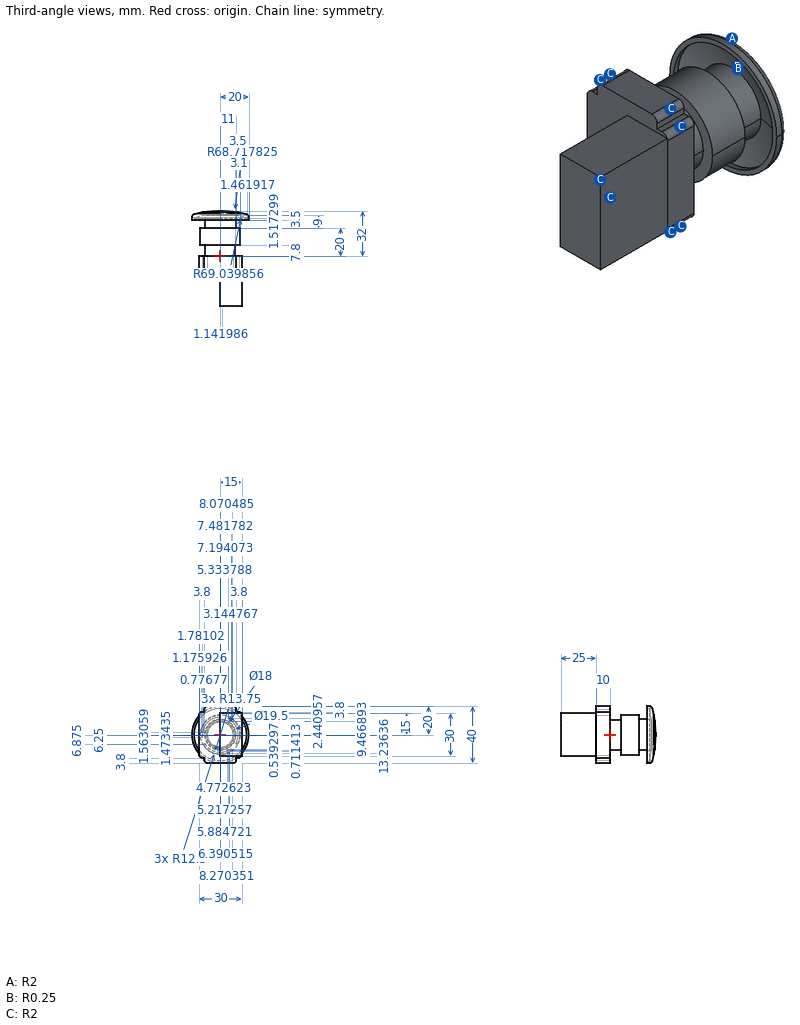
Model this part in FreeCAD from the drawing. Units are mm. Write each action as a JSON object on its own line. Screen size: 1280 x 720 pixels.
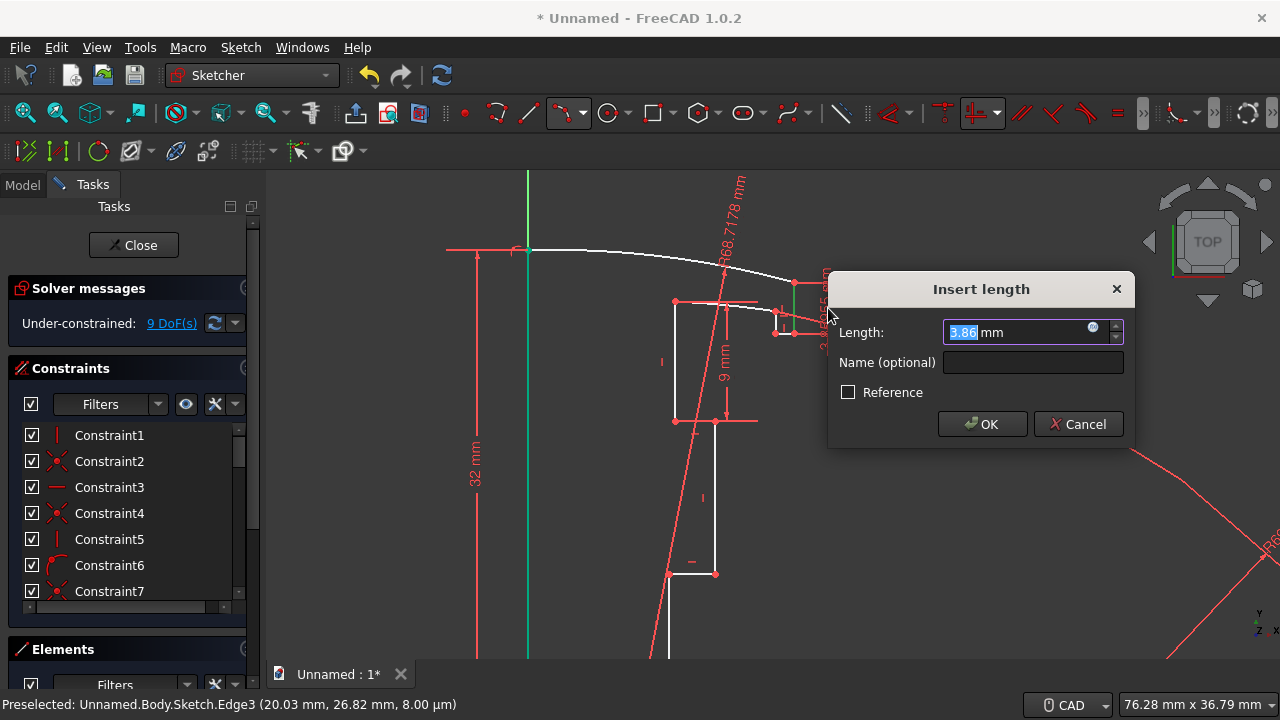
{"action": "type", "text": "3.5"}
{"action": "key", "text": "Return"}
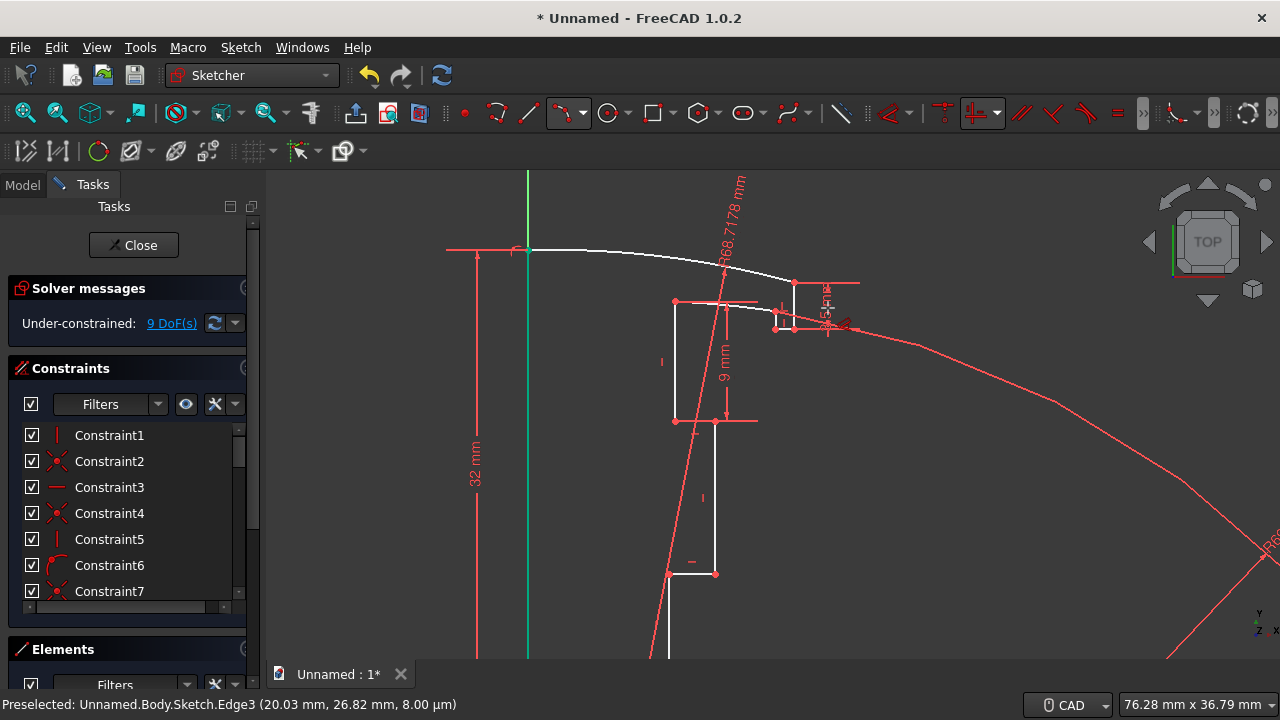
{"action": "left_click", "coordinate": [669, 604]}
{"action": "left_click", "coordinate": [703, 603]}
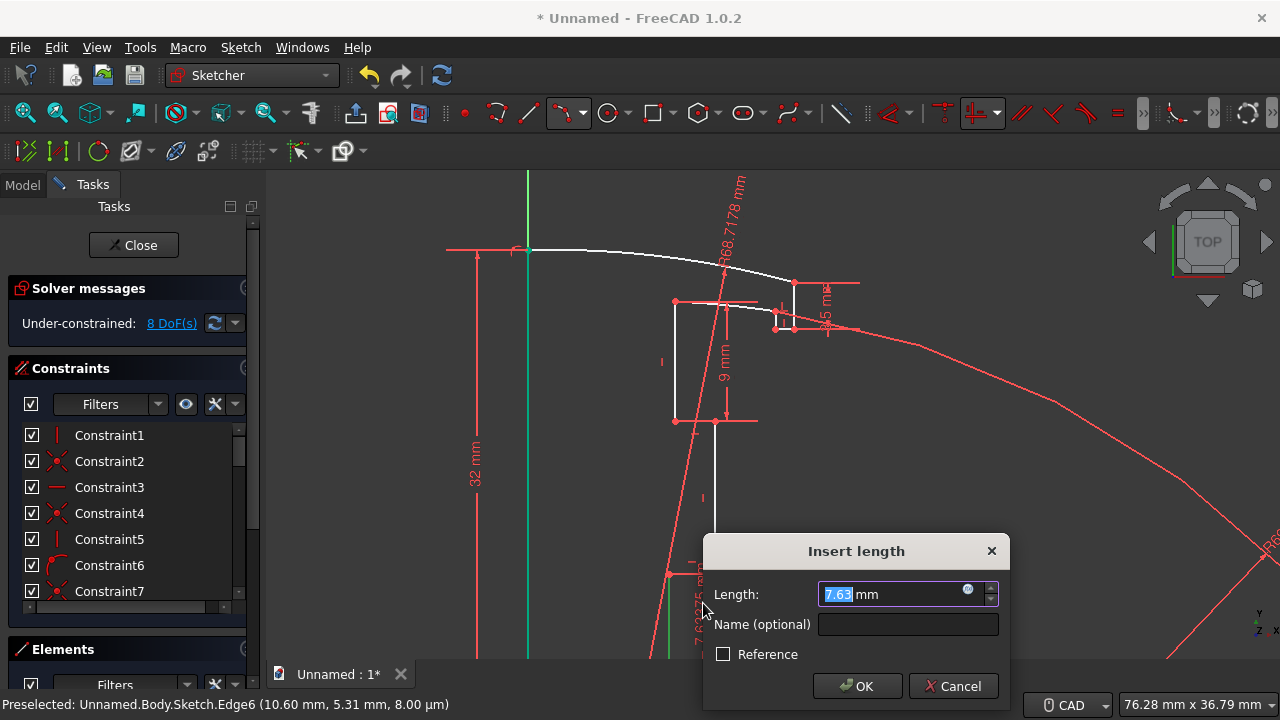
{"action": "type", "text": "7.8"}
{"action": "key", "text": "Return"}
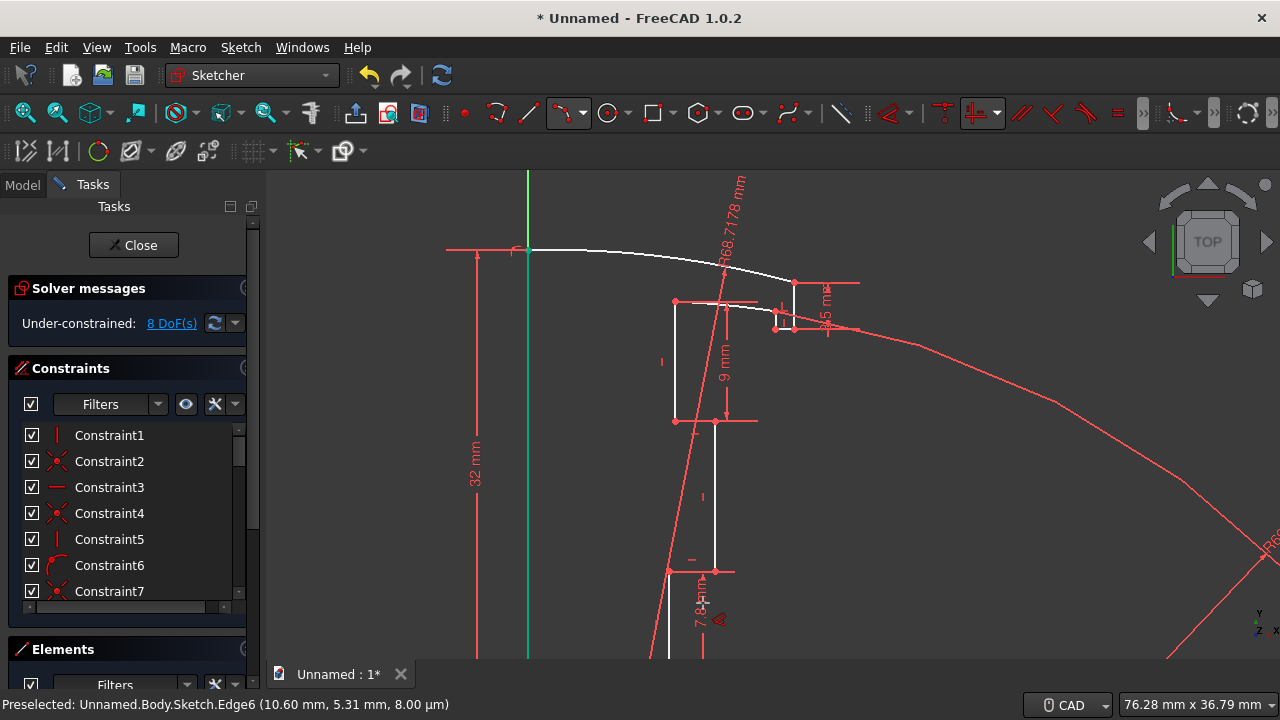
{"action": "left_click", "coordinate": [683, 572]}
{"action": "left_click", "coordinate": [692, 538]}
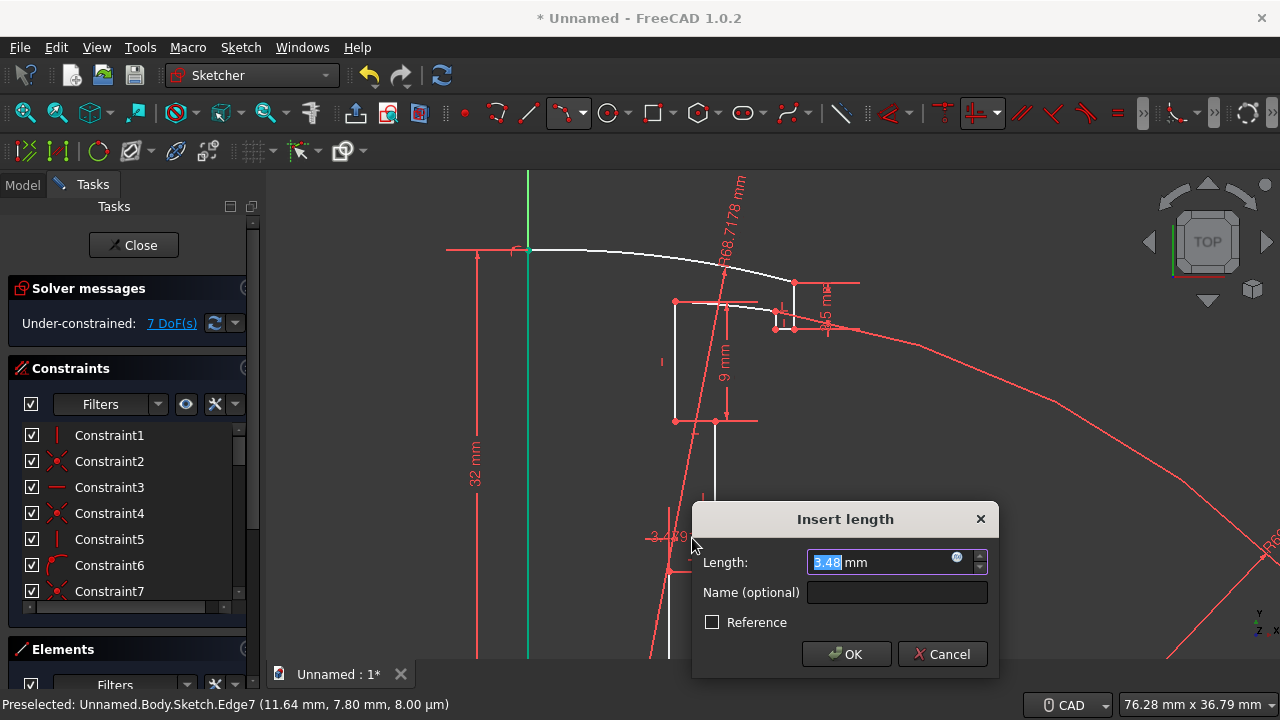
{"action": "type", "text": "3.5"}
{"action": "key", "text": "Return"}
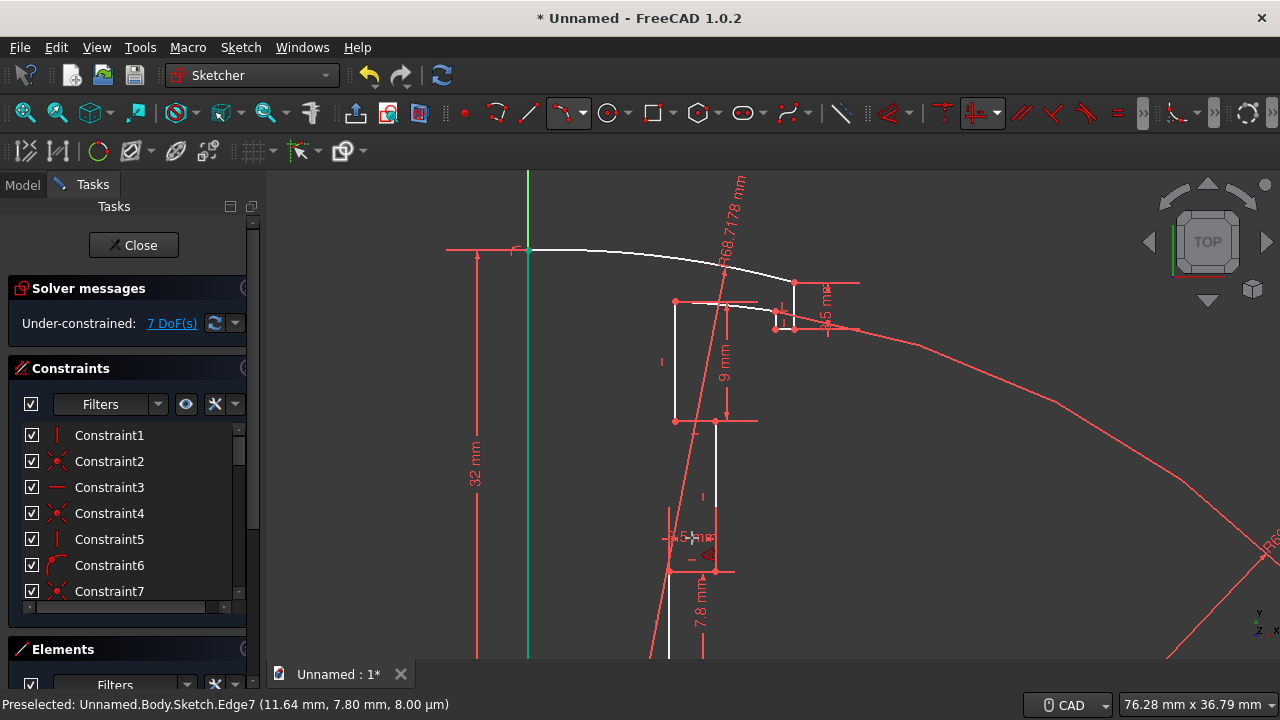
{"action": "left_click", "coordinate": [703, 421]}
{"action": "left_click", "coordinate": [695, 387]}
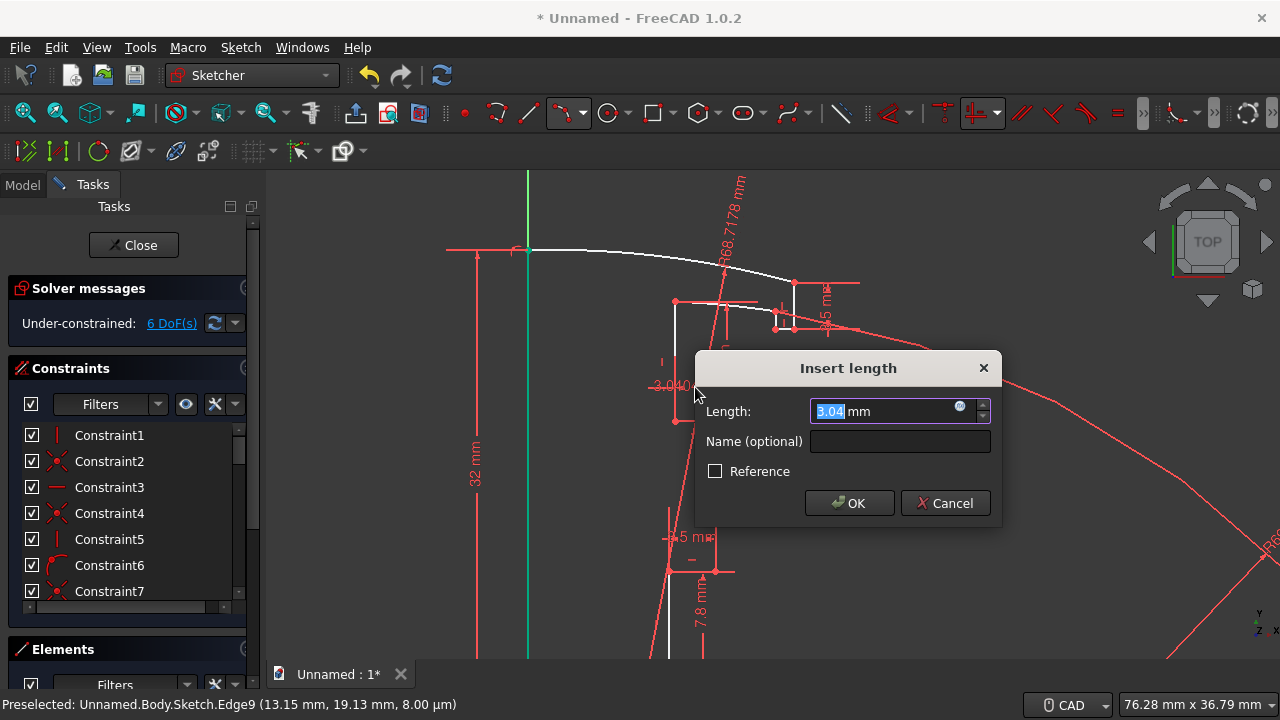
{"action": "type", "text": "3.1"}
{"action": "key", "text": "Return"}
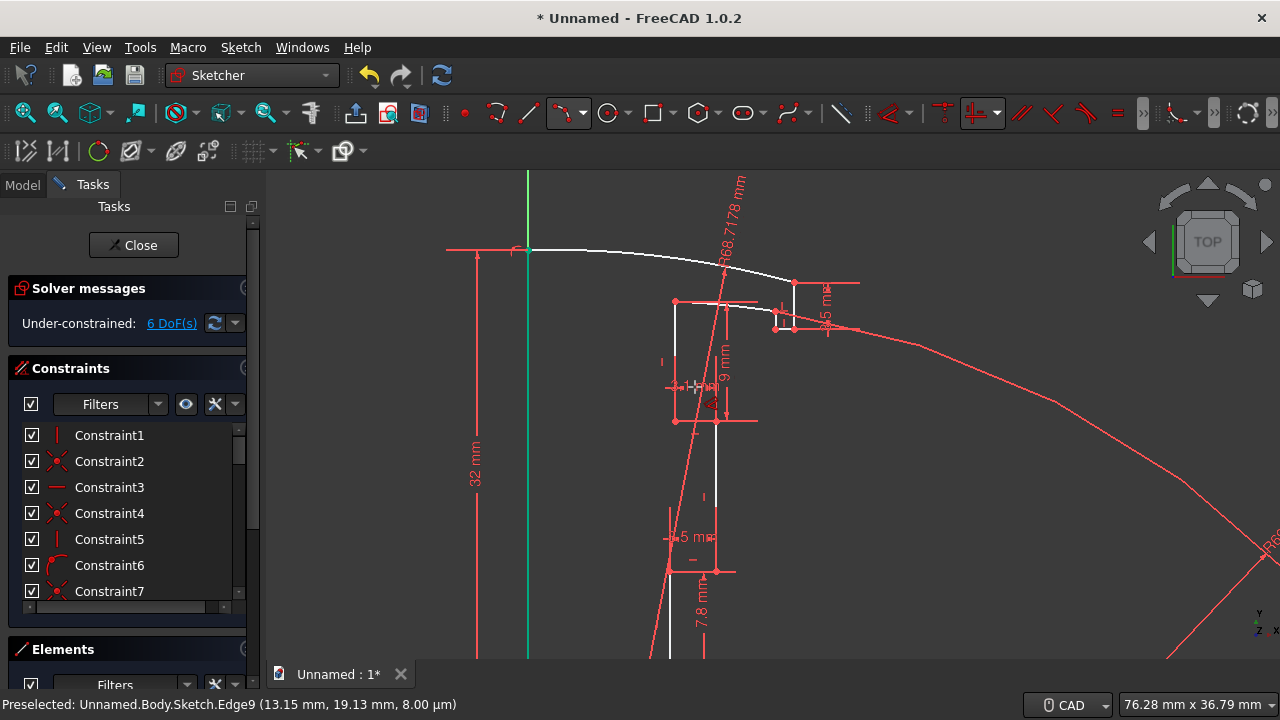
{"action": "left_click", "coordinate": [794, 329]}
{"action": "left_click", "coordinate": [661, 295]}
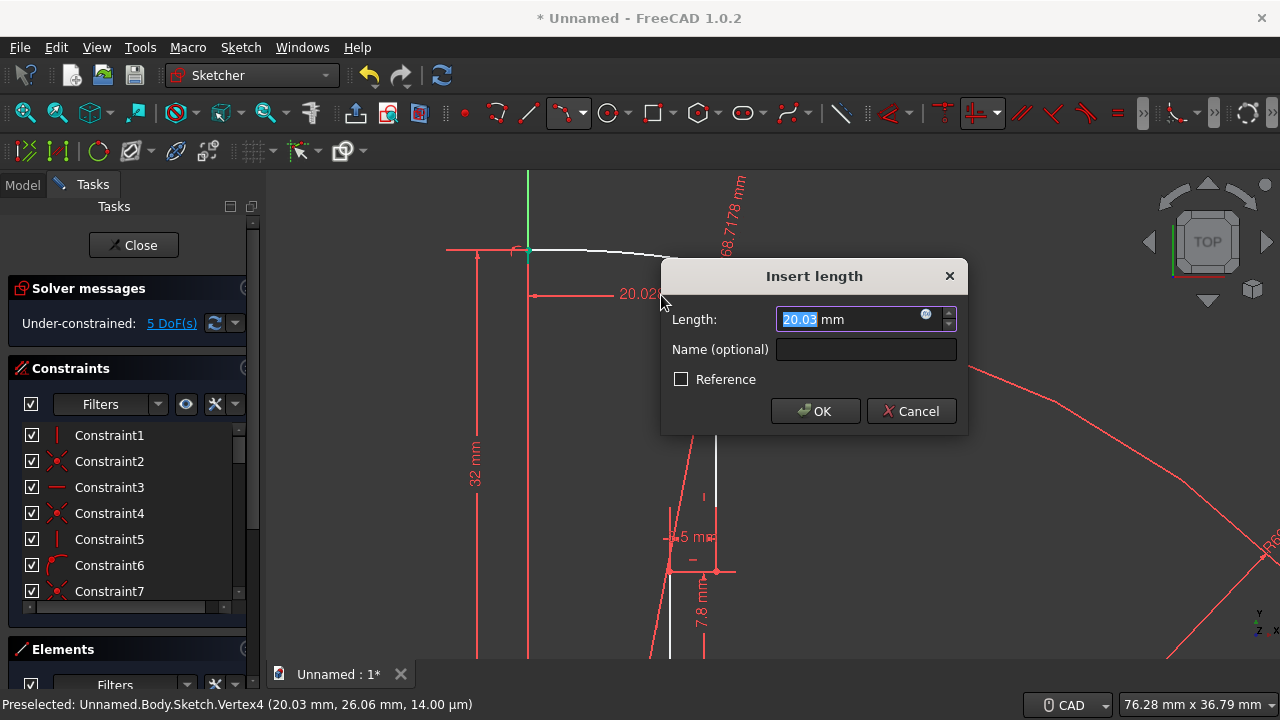
{"action": "type", "text": "20"}
{"action": "key", "text": "Return"}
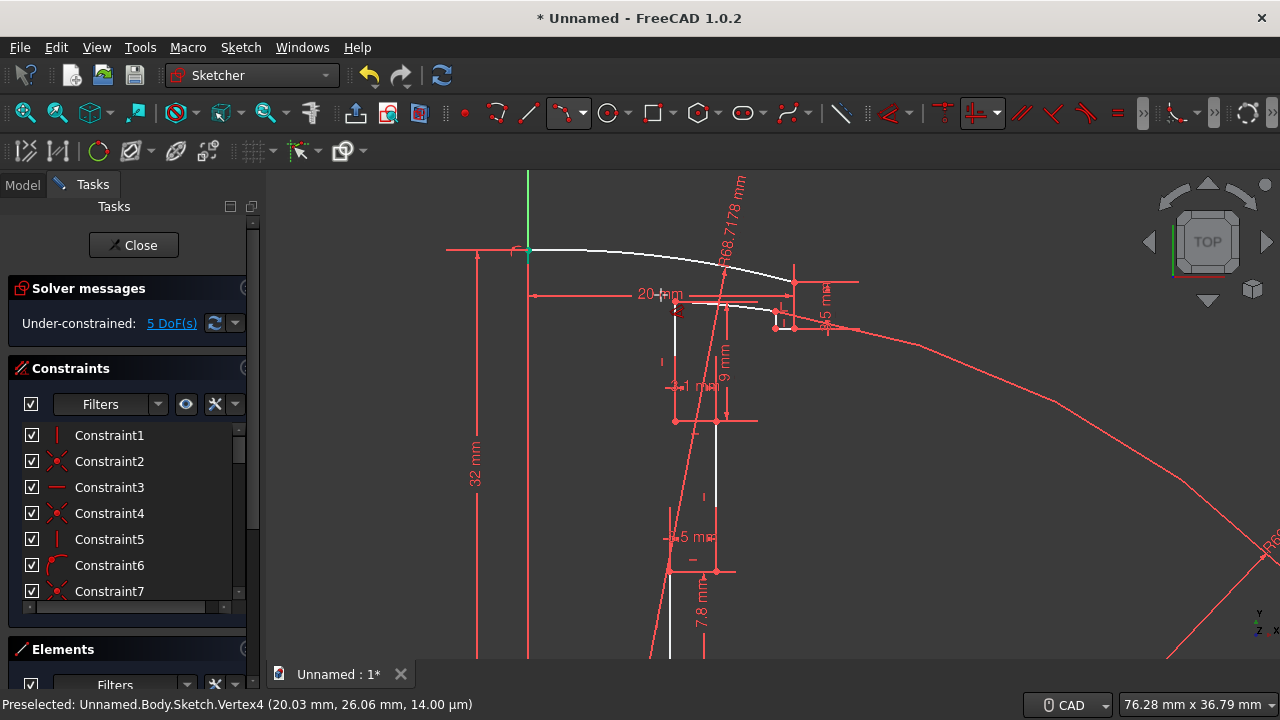
{"action": "left_click", "coordinate": [716, 421]}
{"action": "left_click", "coordinate": [494, 526]}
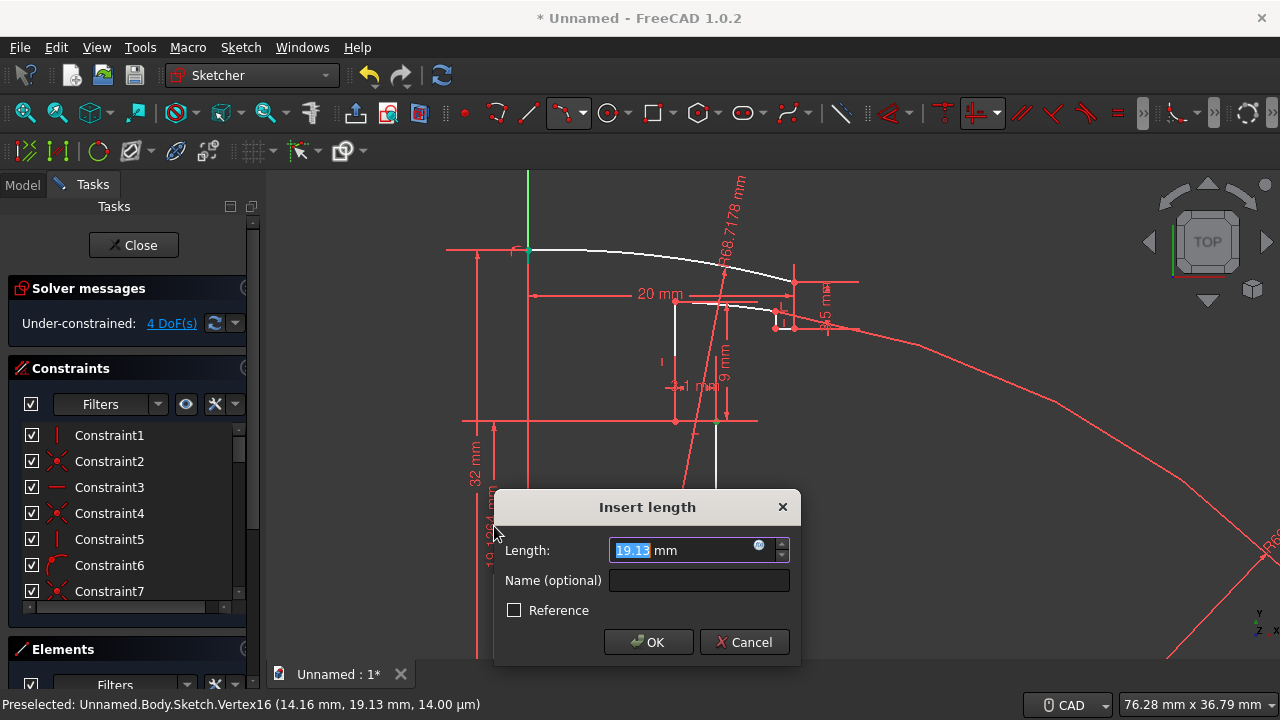
{"action": "type", "text": "20"}
{"action": "key", "text": "Return"}